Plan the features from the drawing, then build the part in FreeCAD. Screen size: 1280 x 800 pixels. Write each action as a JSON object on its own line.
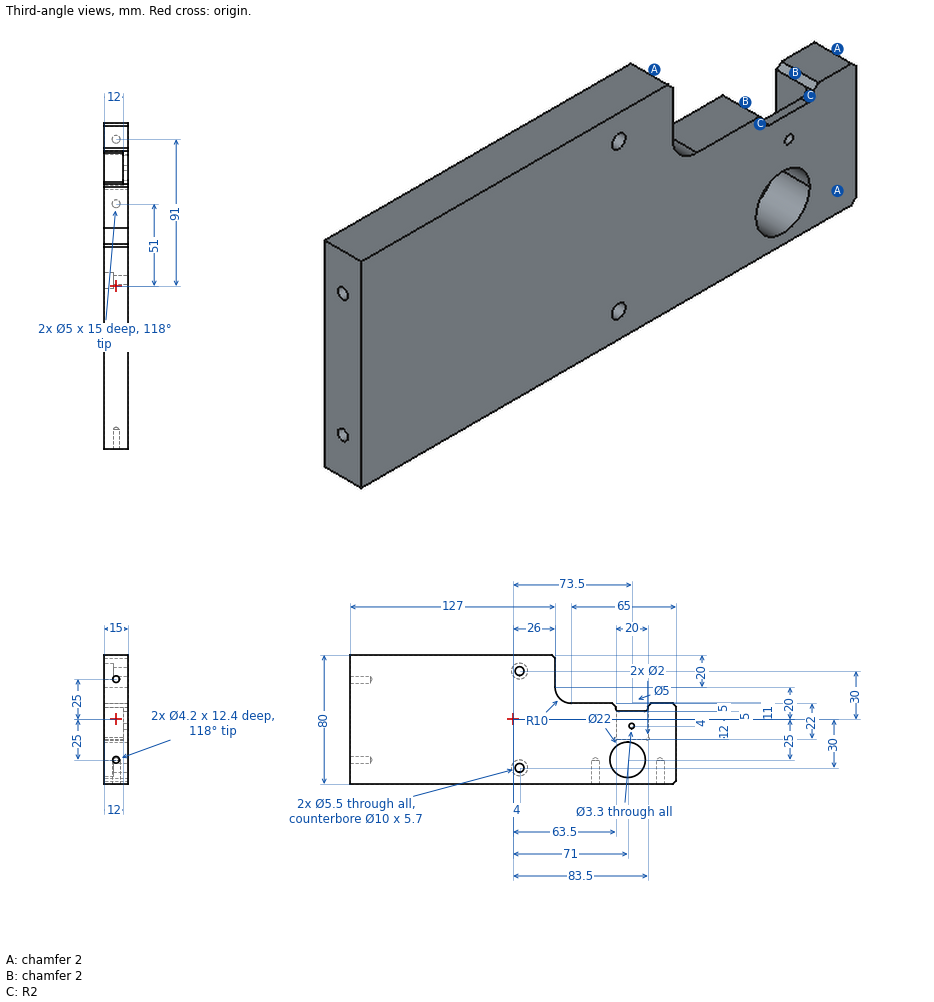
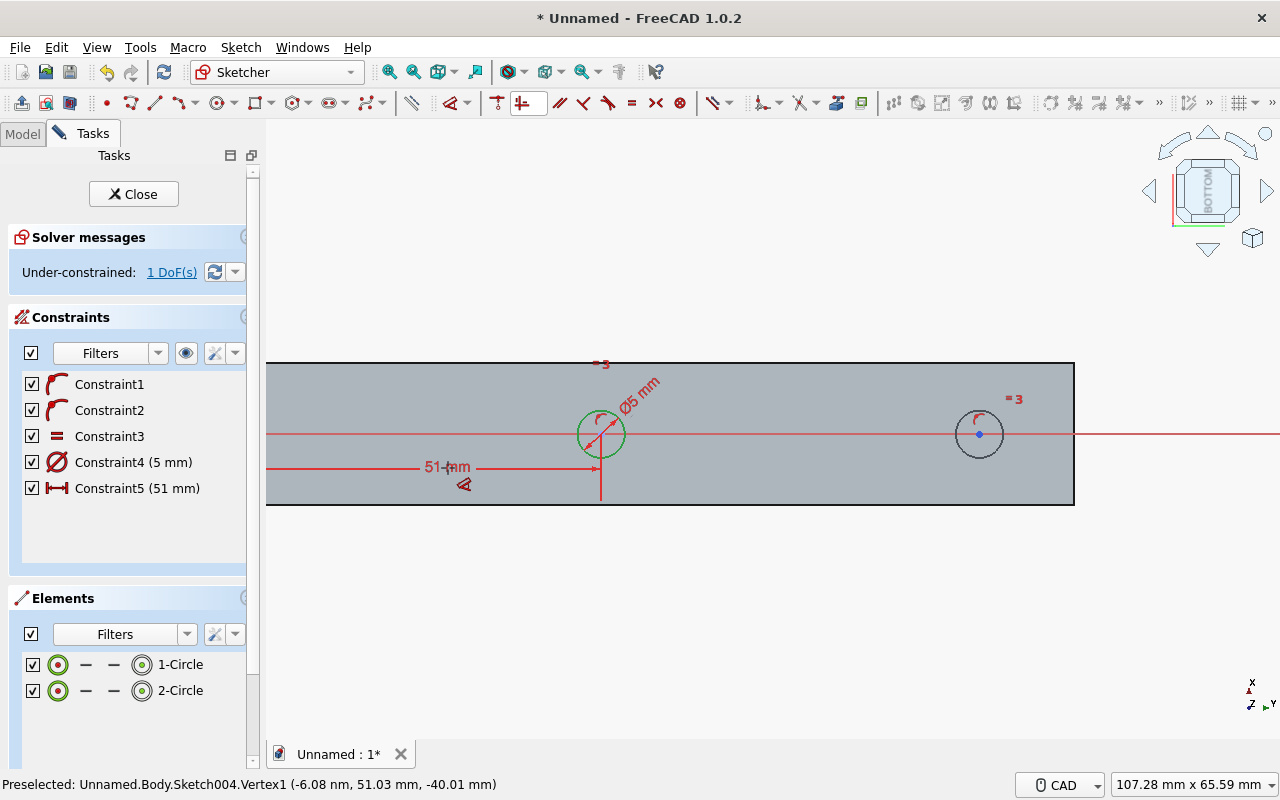
{"action": "left_click", "coordinate": [980, 434]}
{"action": "left_click", "coordinate": [637, 468]}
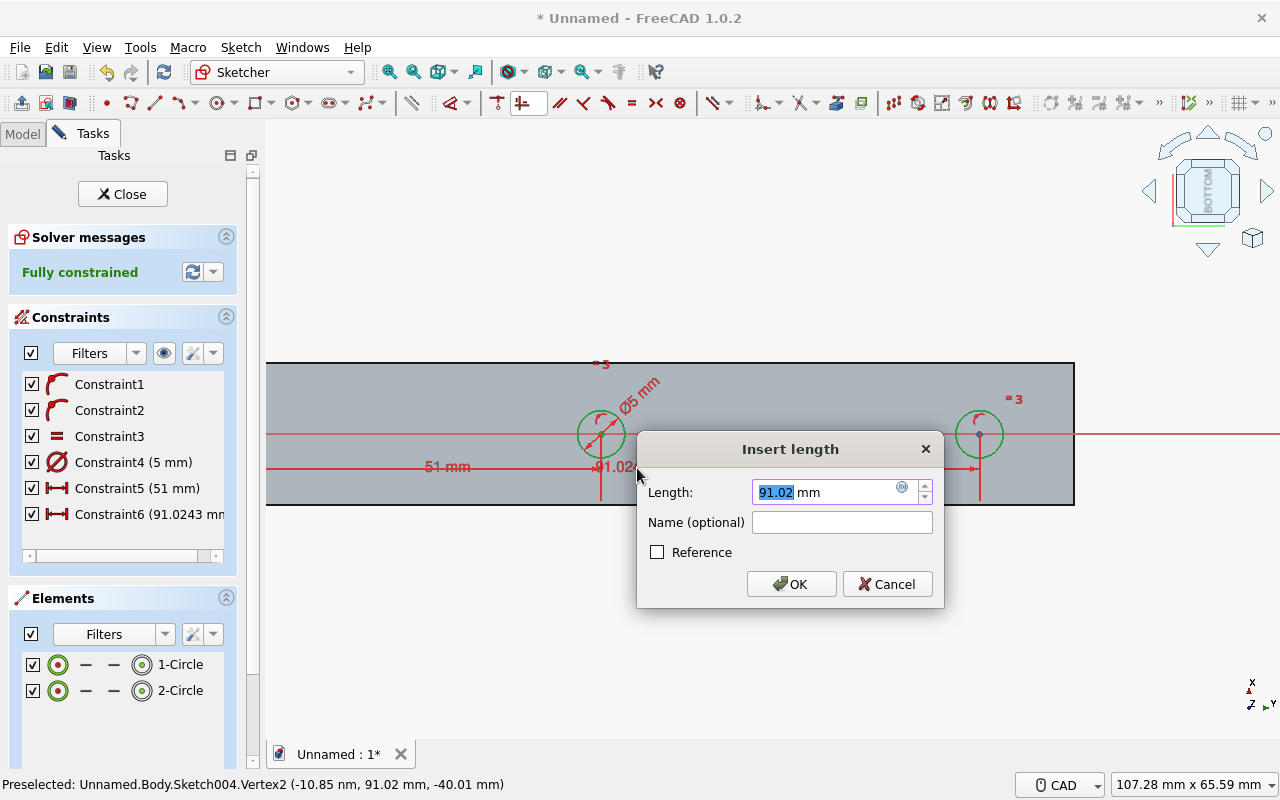
{"action": "type", "text": "91"}
{"action": "key", "text": "Return"}
{"action": "key", "text": "Escape"}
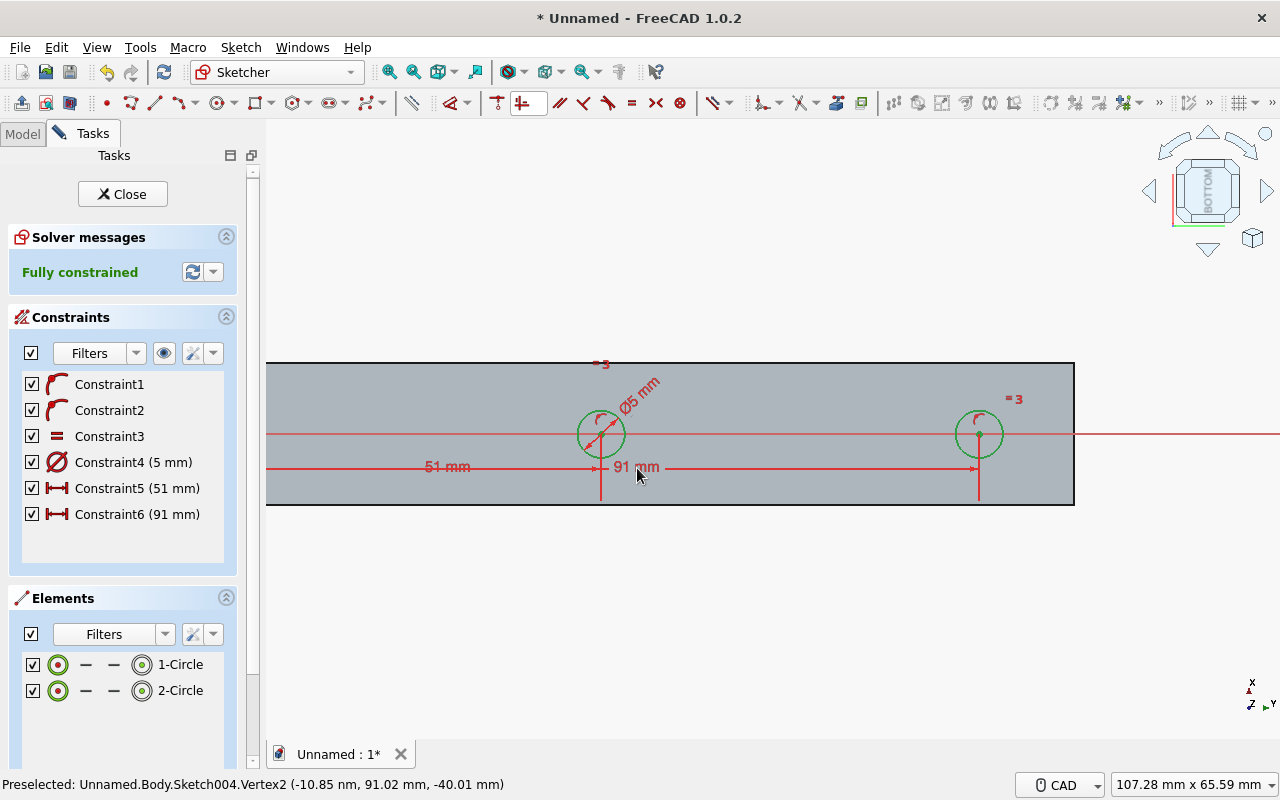
{"action": "left_click", "coordinate": [123, 194]}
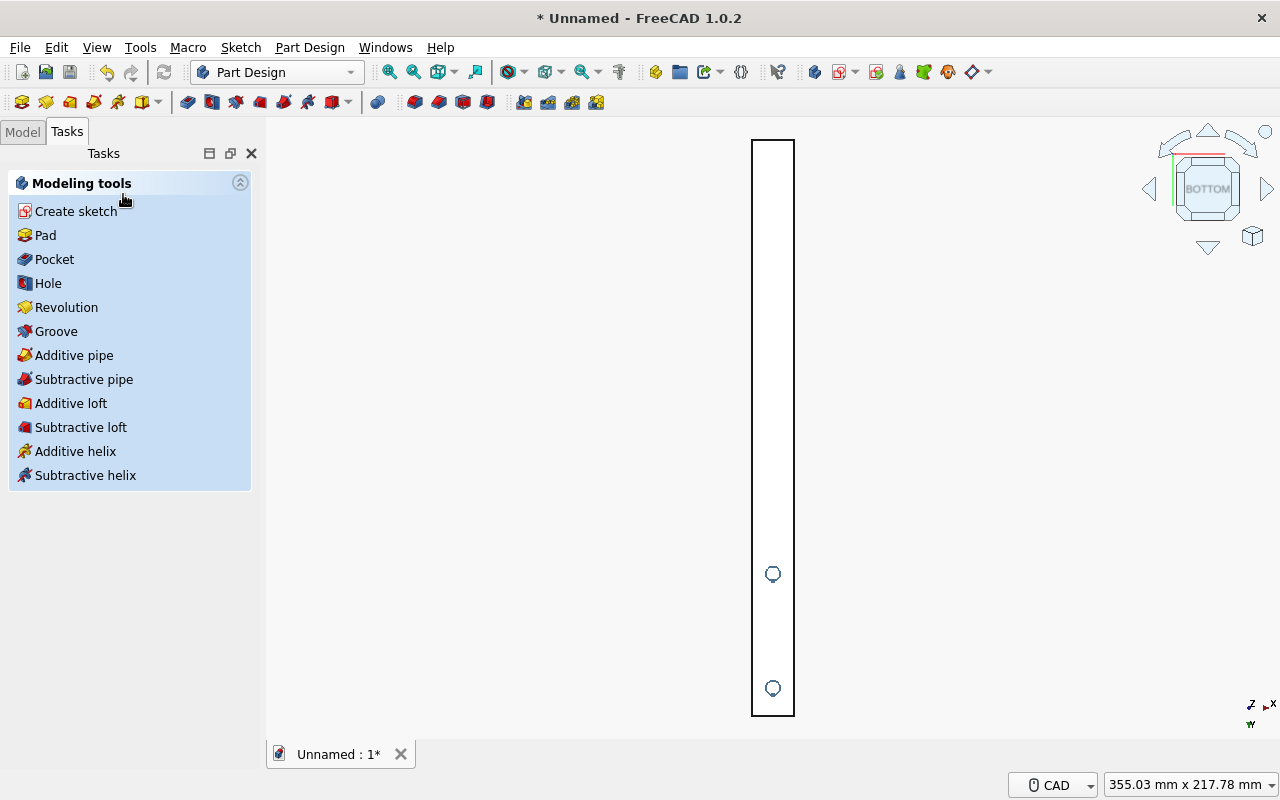
{"action": "left_click", "coordinate": [212, 102]}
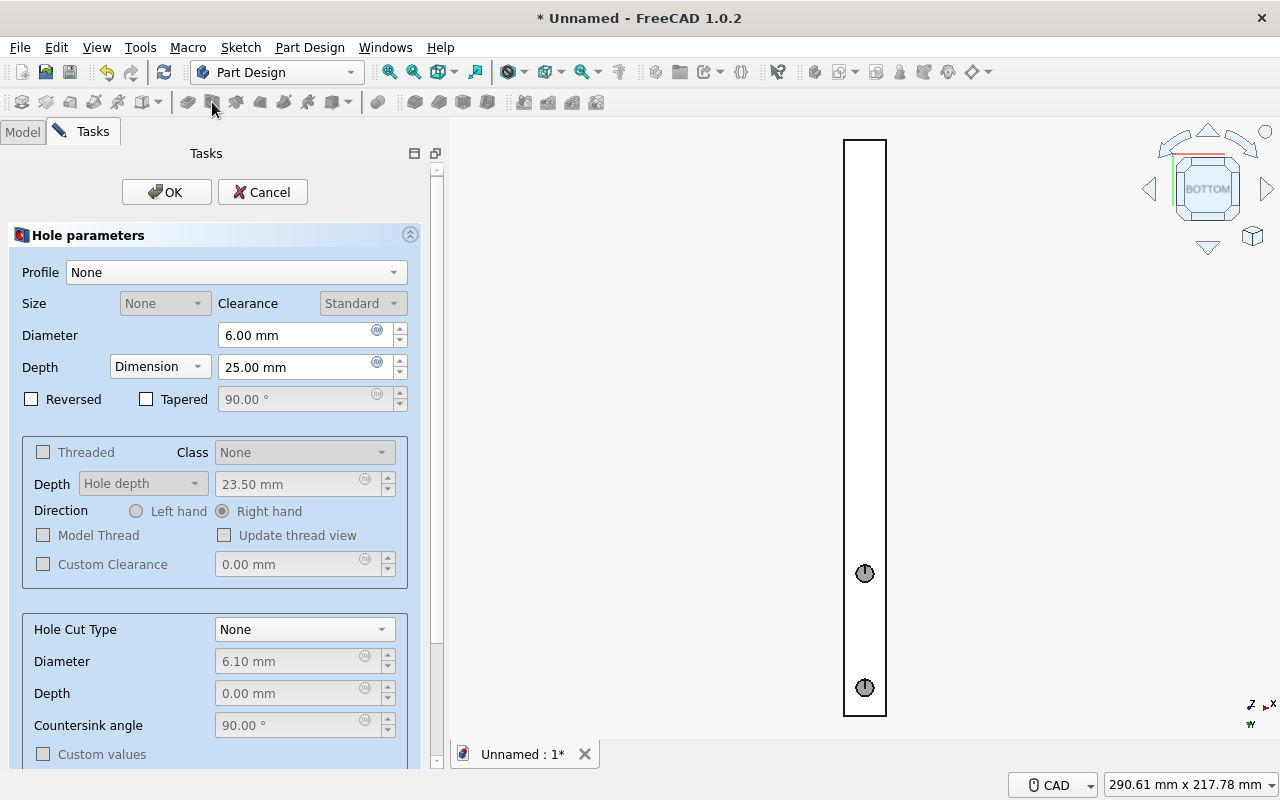
{"action": "triple_click", "coordinate": [305, 335]}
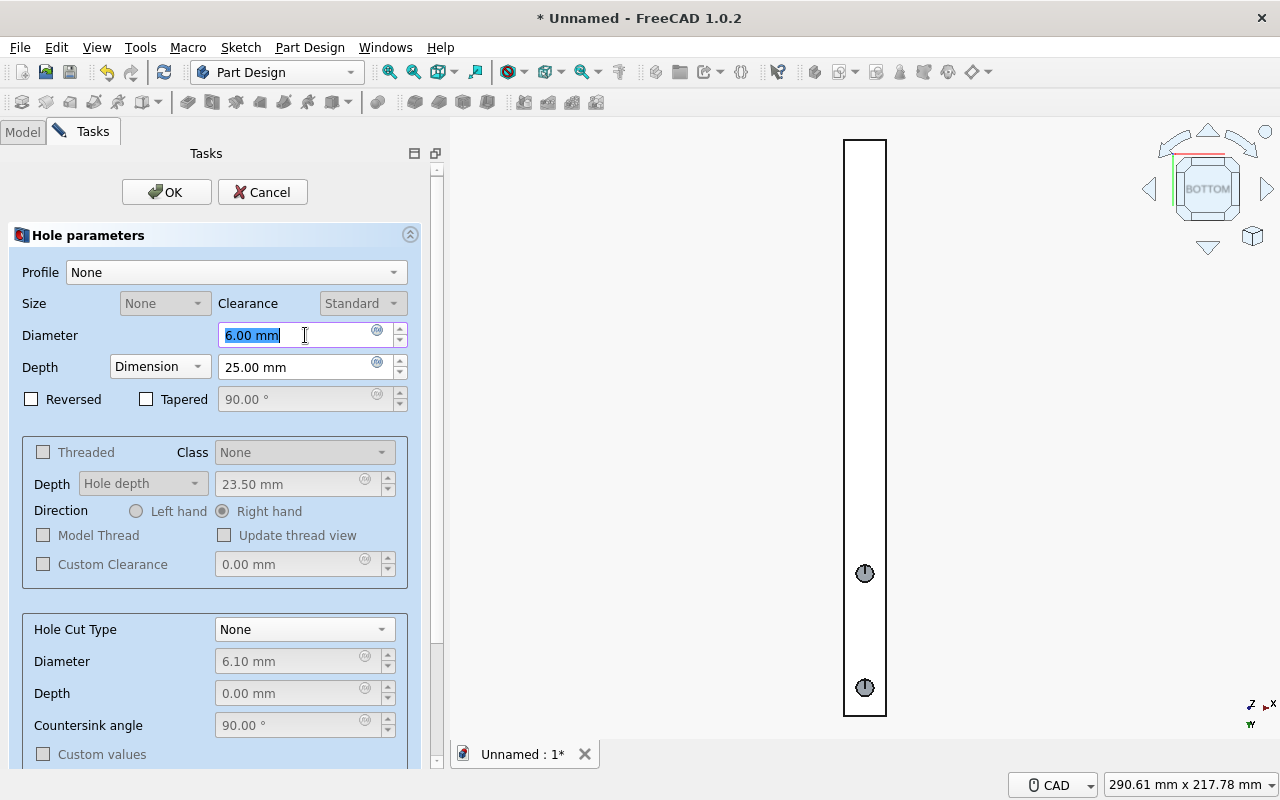
{"action": "type", "text": "5"}
{"action": "key", "text": "Tab"}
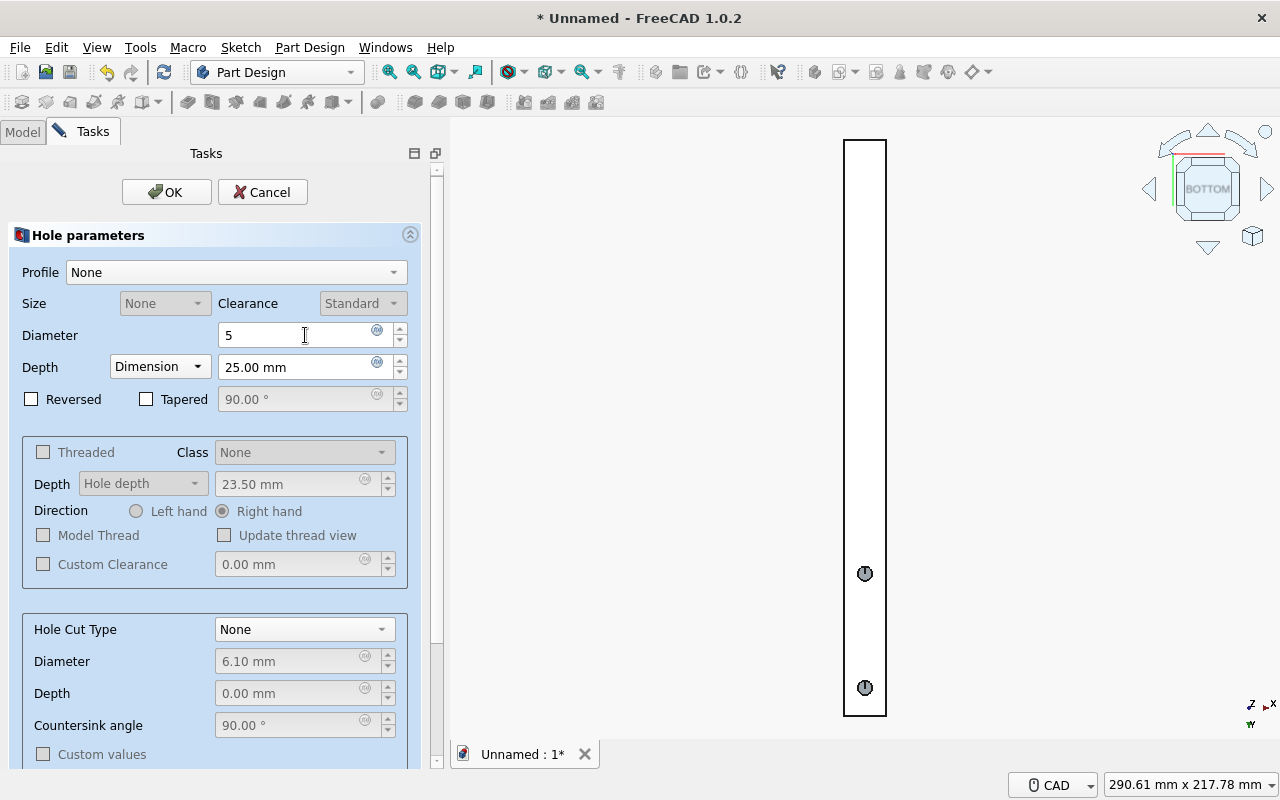
{"action": "triple_click", "coordinate": [305, 367]}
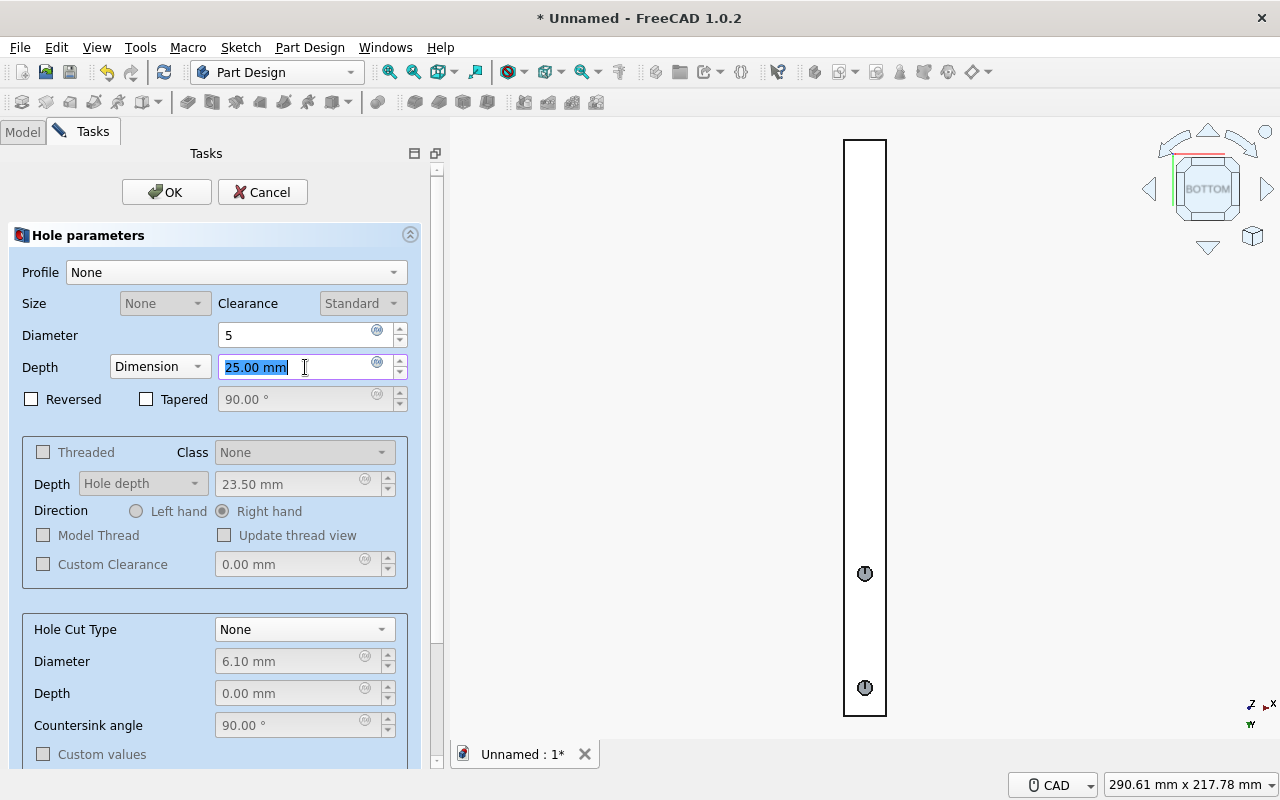
{"action": "type", "text": "15"}
{"action": "key", "text": "Tab"}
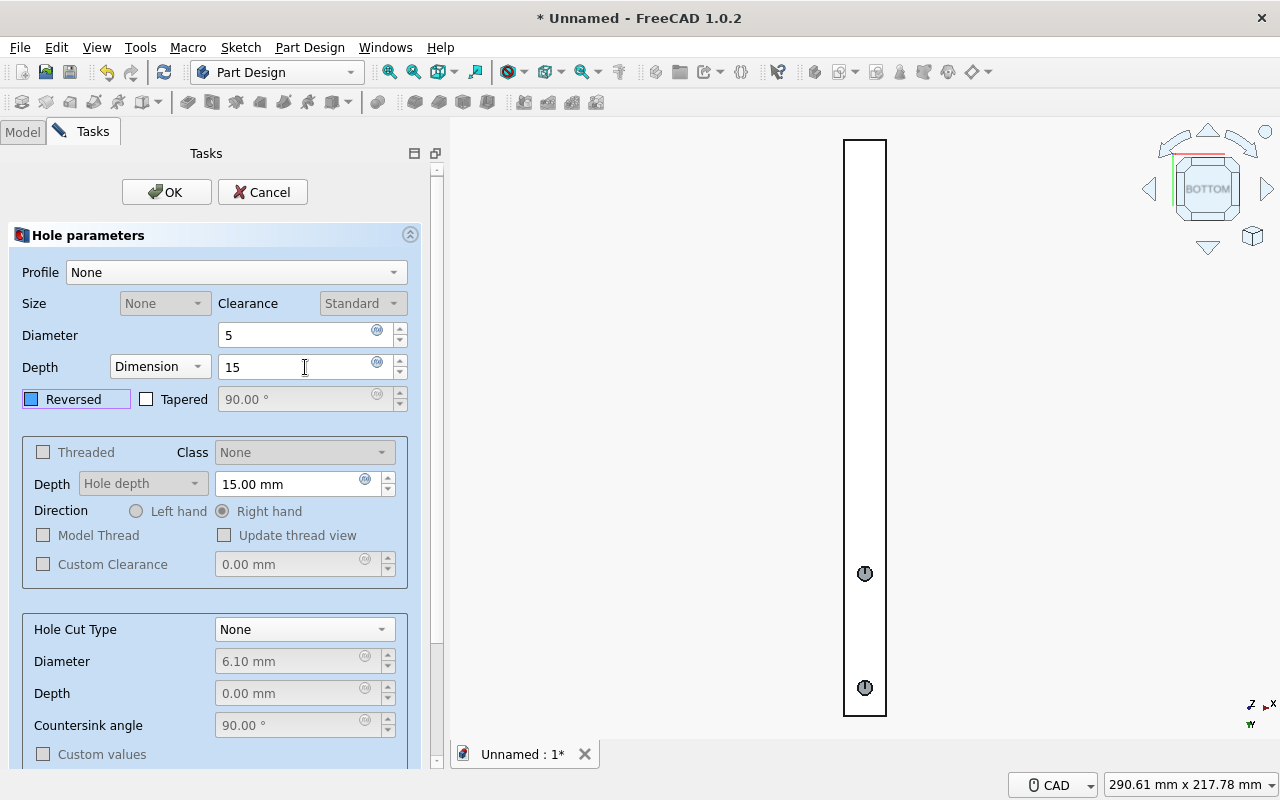
{"action": "left_click", "coordinate": [167, 192]}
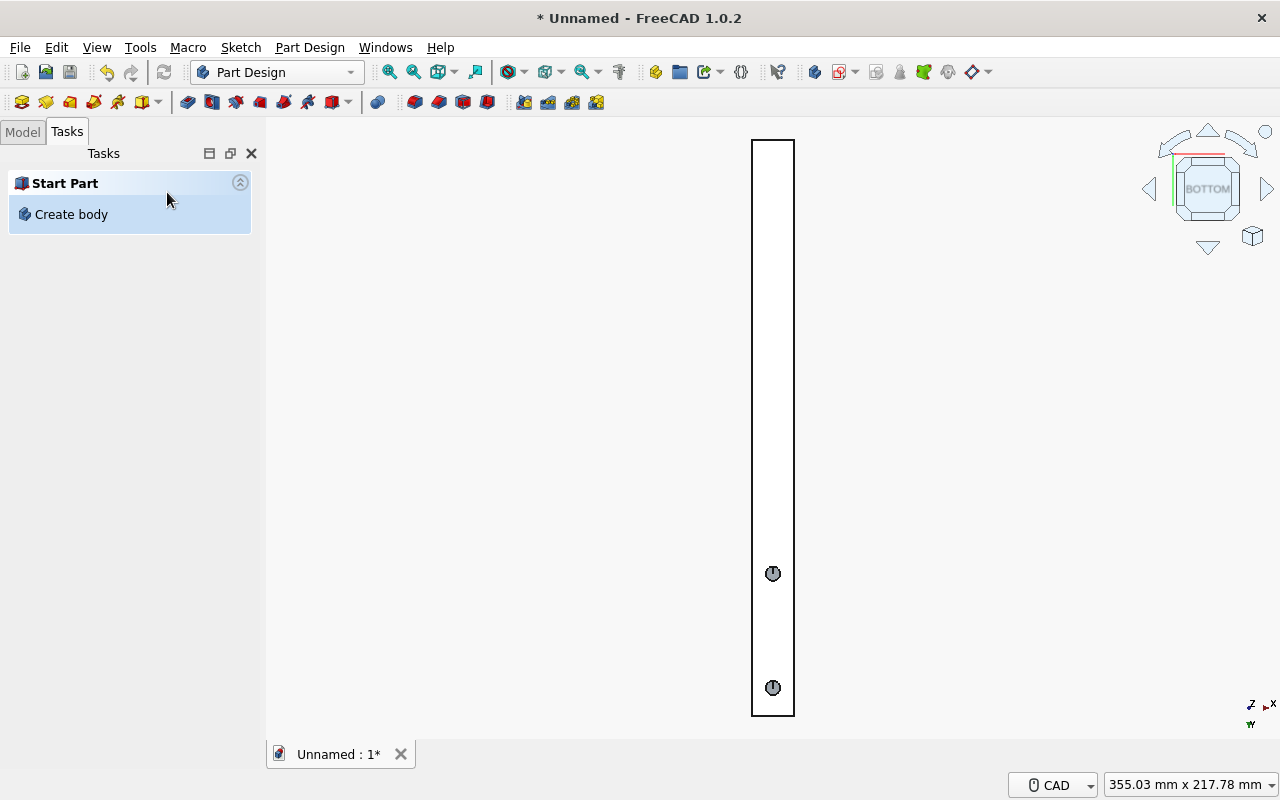
{"action": "key", "text": "0"}